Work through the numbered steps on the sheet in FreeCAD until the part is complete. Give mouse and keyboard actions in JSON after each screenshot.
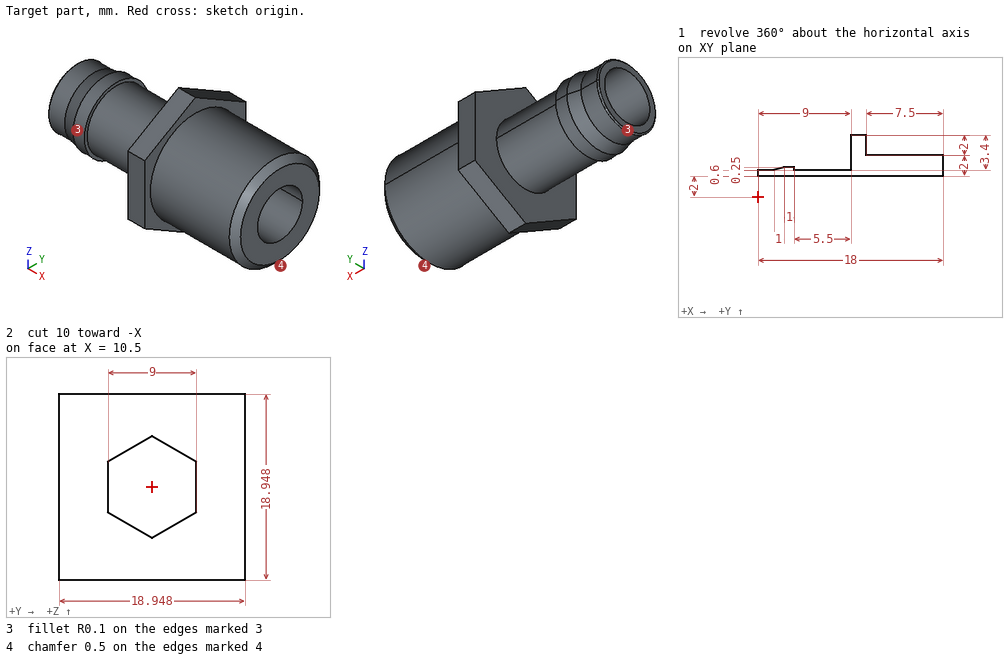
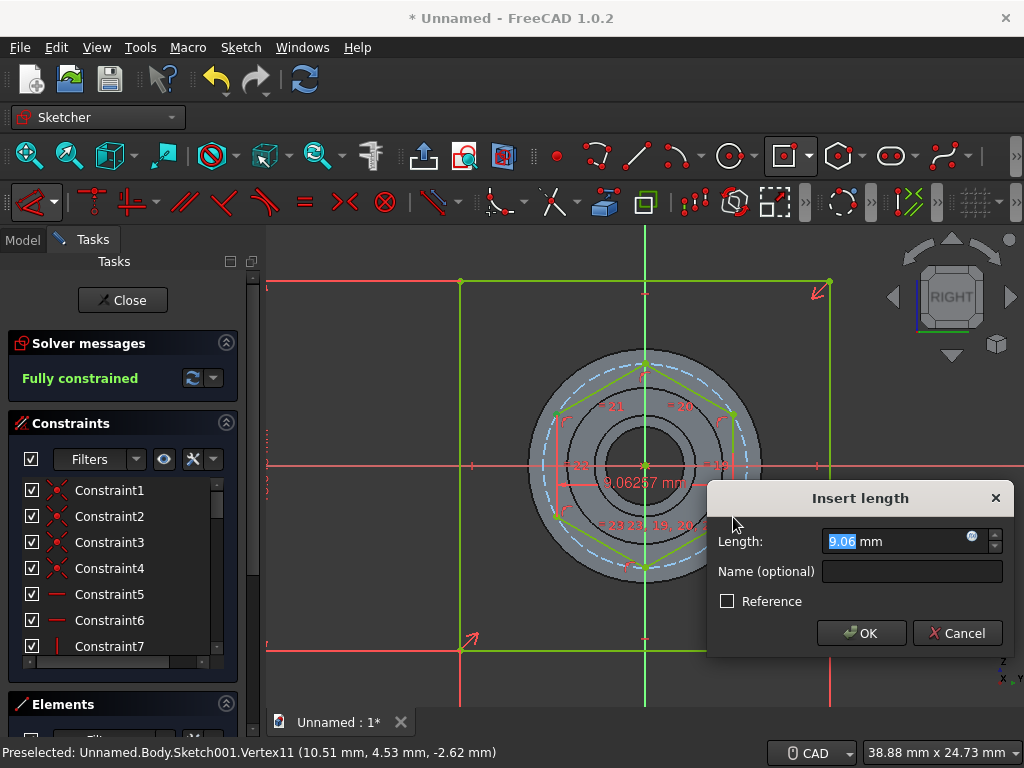
{"action": "type", "text": "9"}
{"action": "key", "text": "Return"}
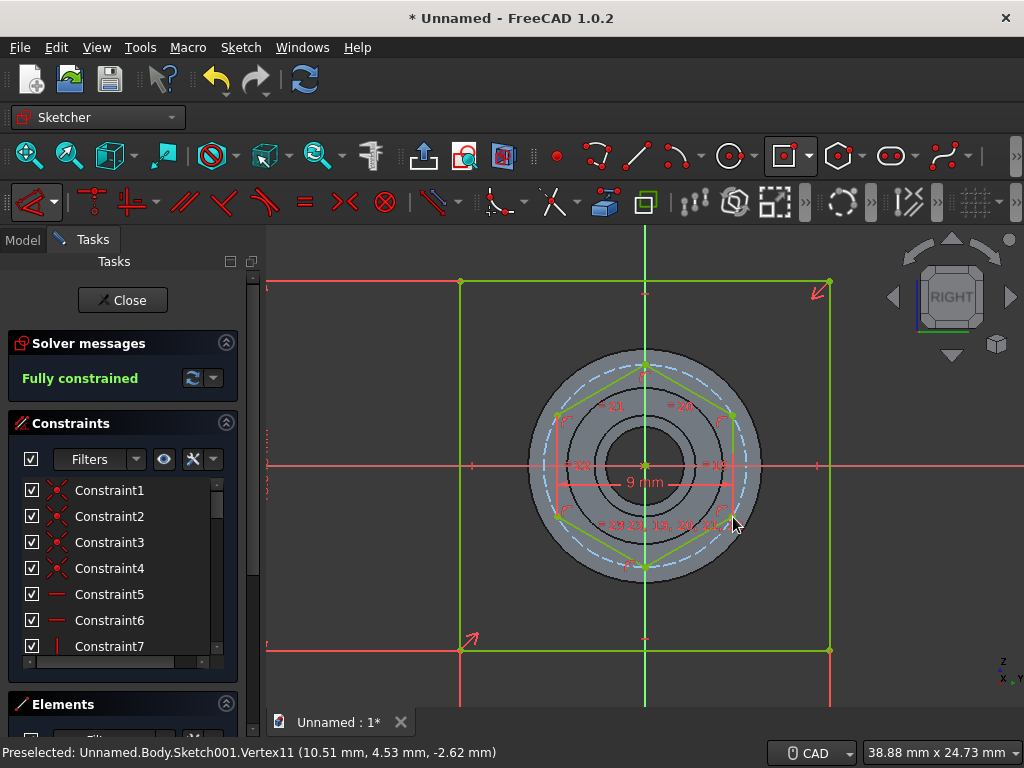
{"action": "left_click", "coordinate": [123, 300]}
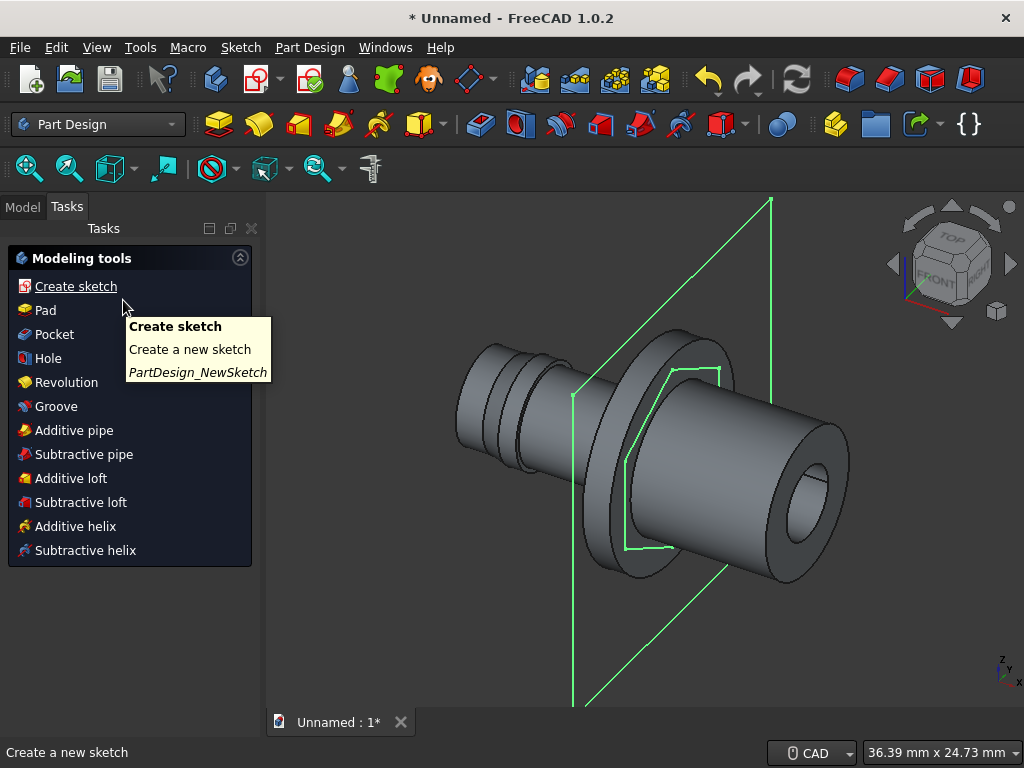
{"action": "left_click", "coordinate": [482, 124]}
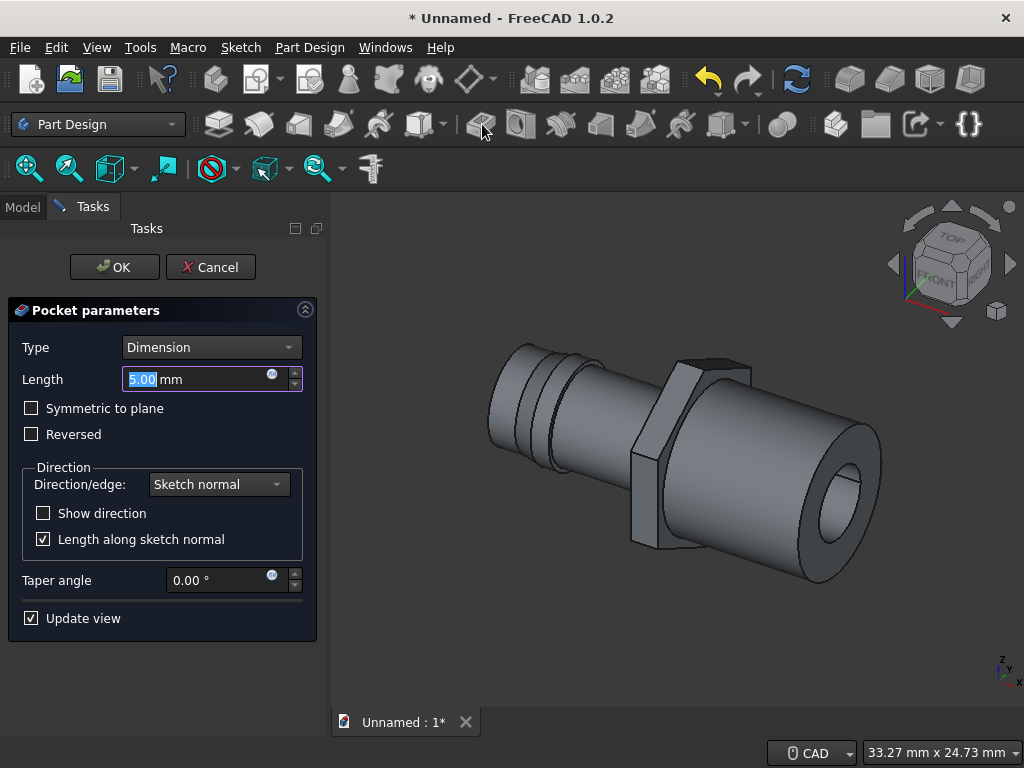
{"action": "type", "text": "10"}
{"action": "key", "text": "Tab"}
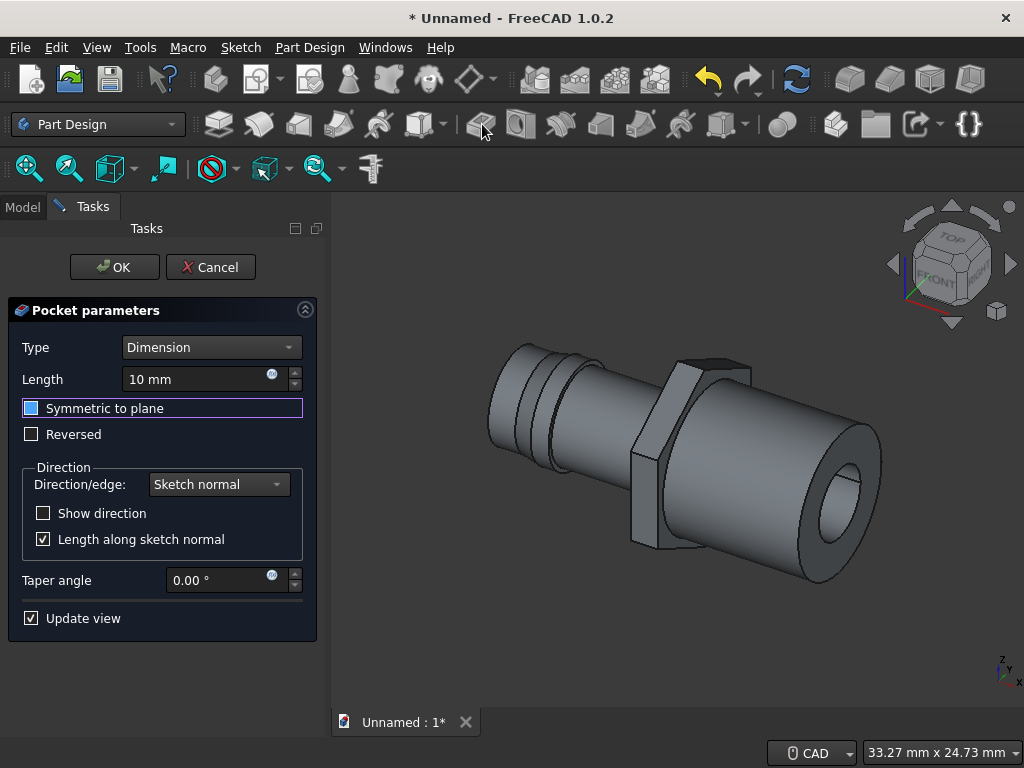
{"action": "left_click", "coordinate": [115, 267]}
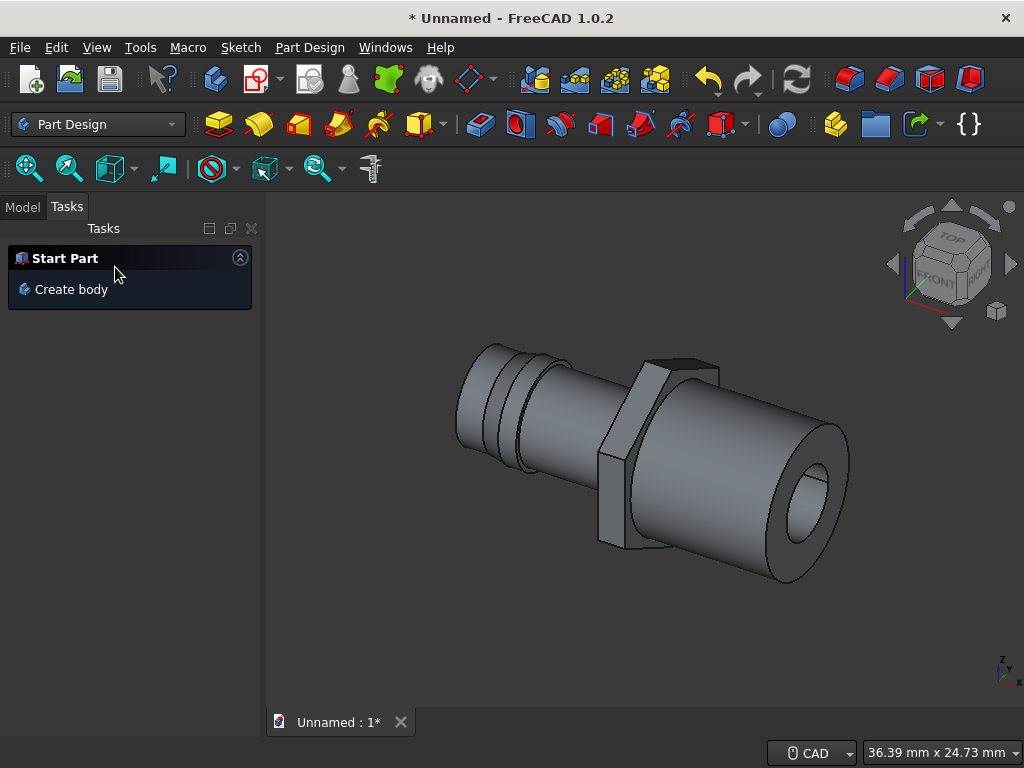
{"action": "left_click", "coordinate": [491, 344]}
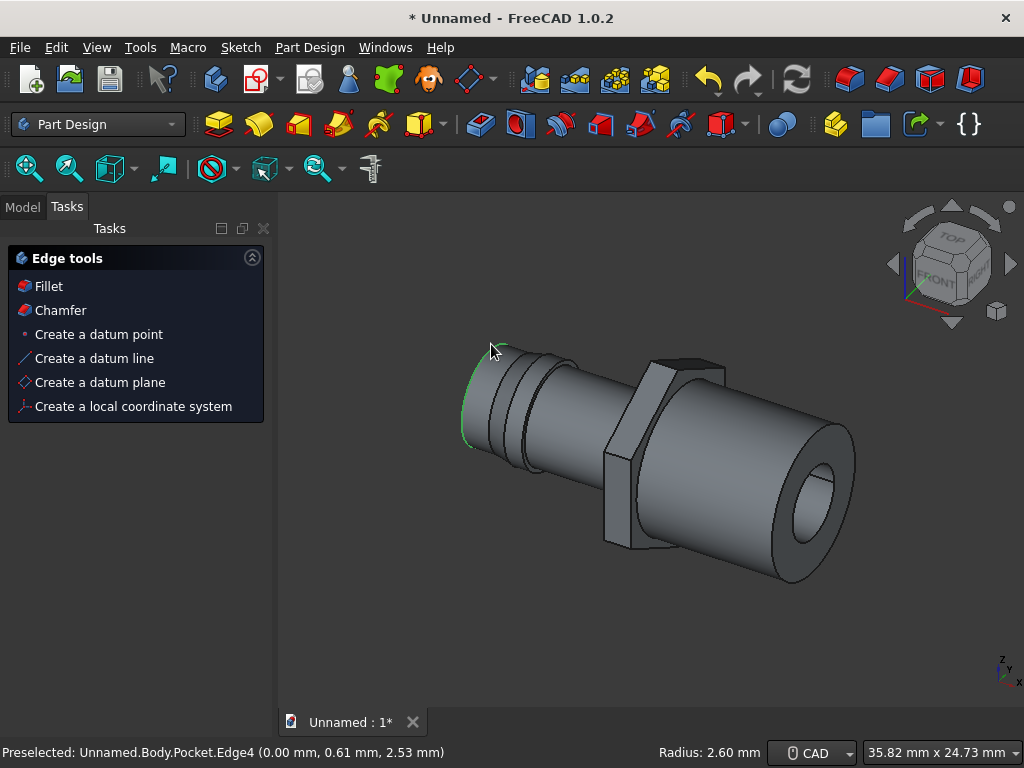
{"action": "left_click", "coordinate": [850, 80]}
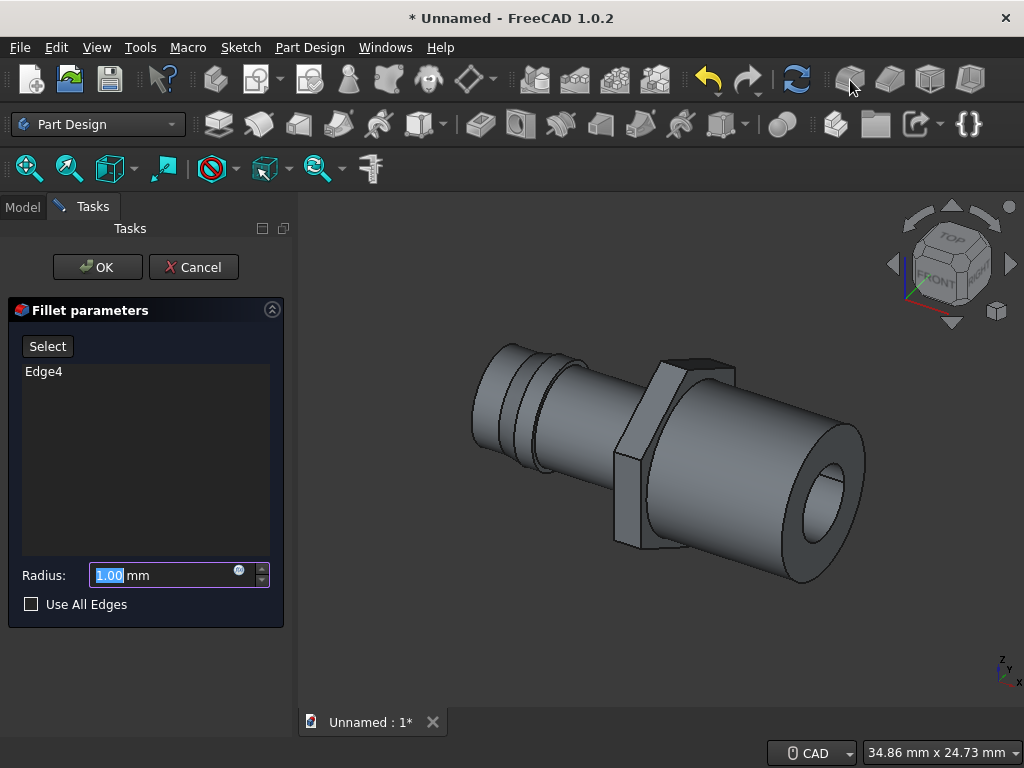
{"action": "type", "text": "0.1"}
{"action": "key", "text": "Tab"}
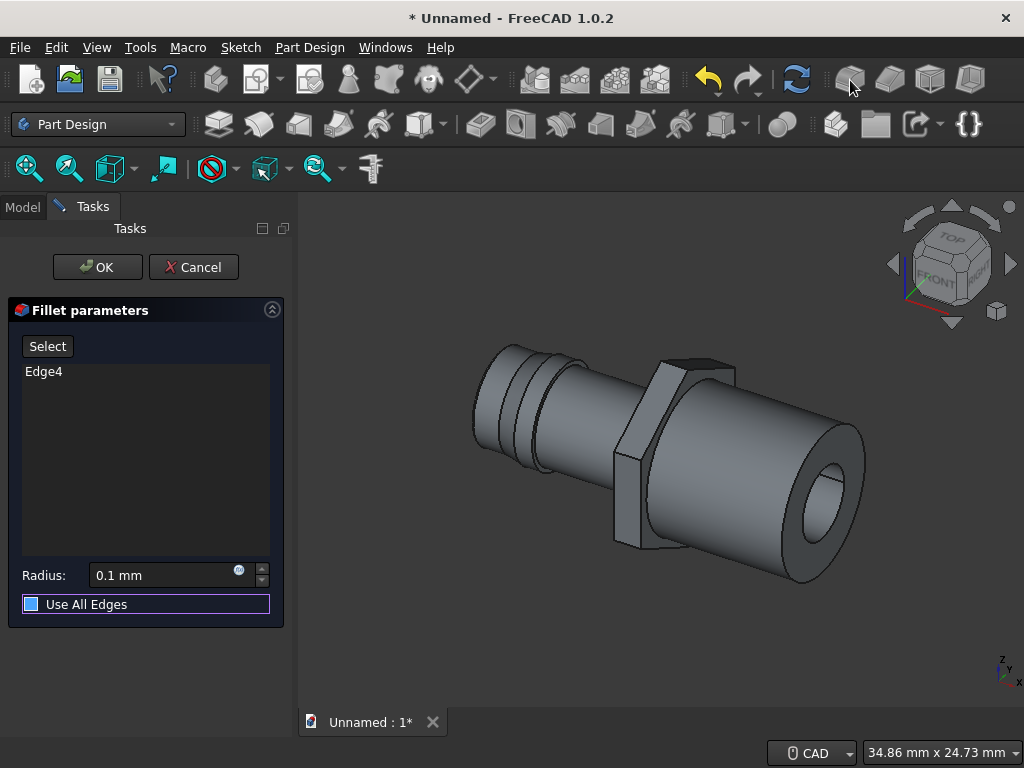
{"action": "left_click", "coordinate": [98, 267]}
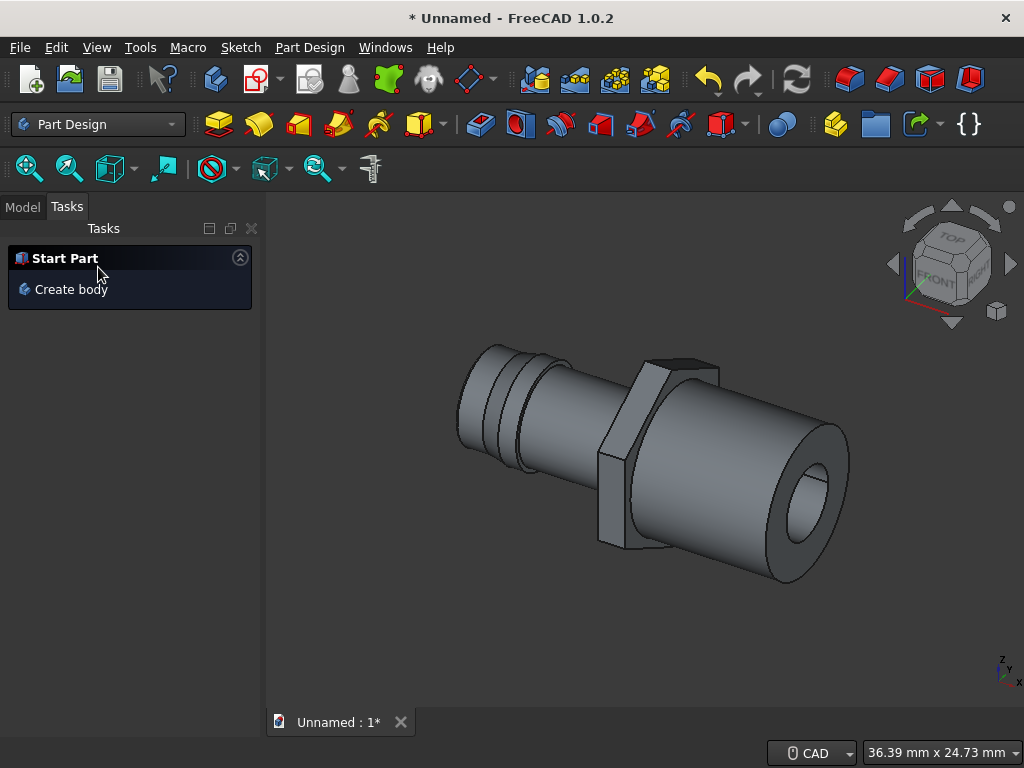
{"action": "left_click", "coordinate": [766, 544]}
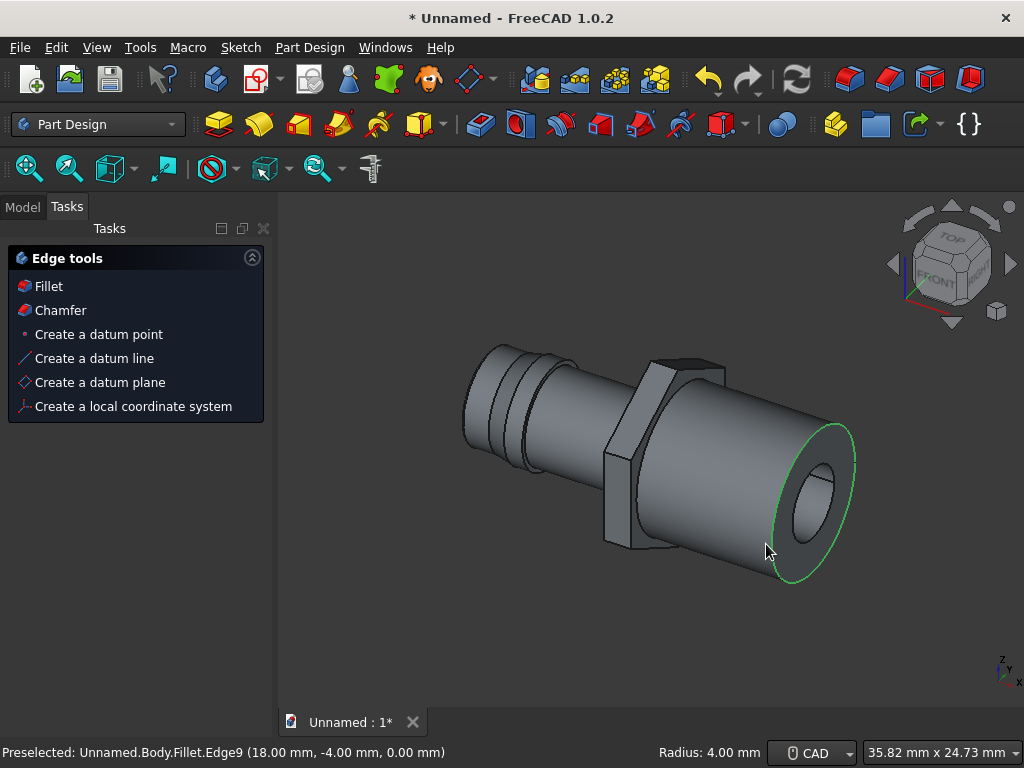
{"action": "left_click", "coordinate": [890, 80]}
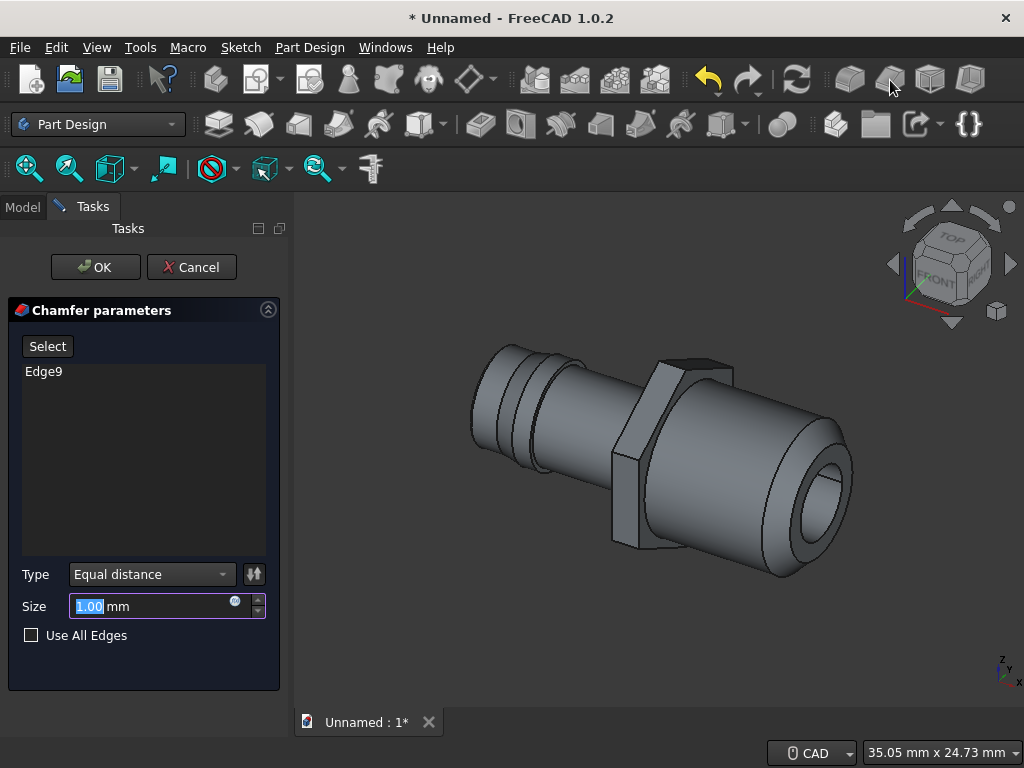
{"action": "type", "text": "0.5"}
{"action": "key", "text": "Tab"}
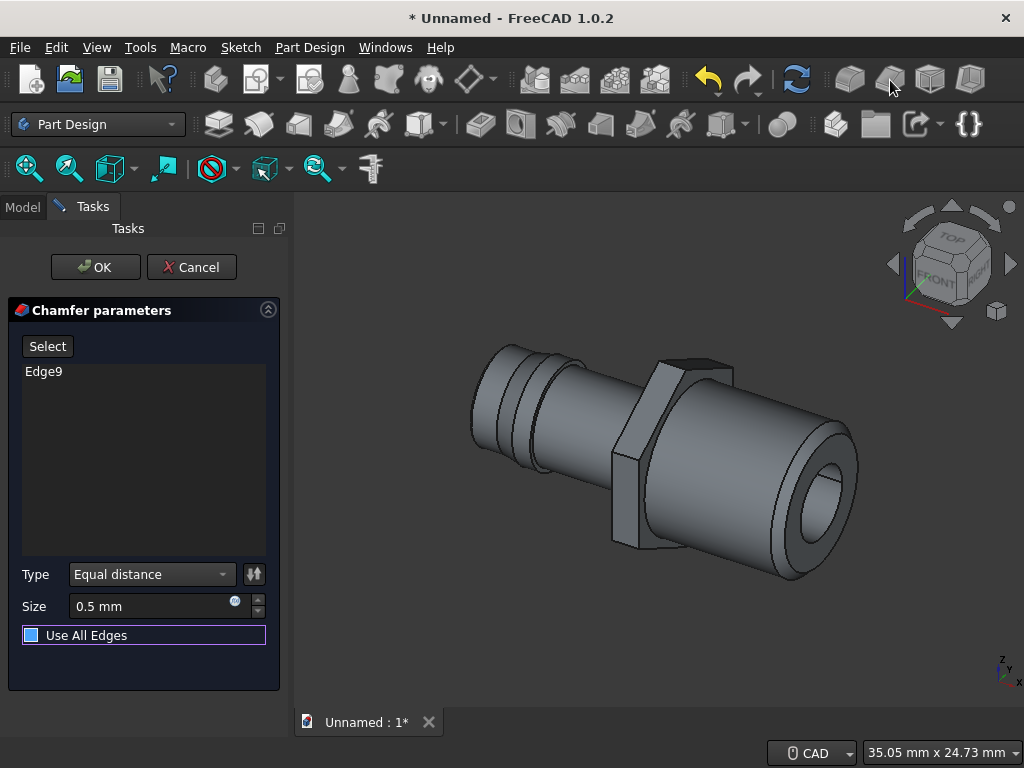
{"action": "left_click", "coordinate": [96, 267]}